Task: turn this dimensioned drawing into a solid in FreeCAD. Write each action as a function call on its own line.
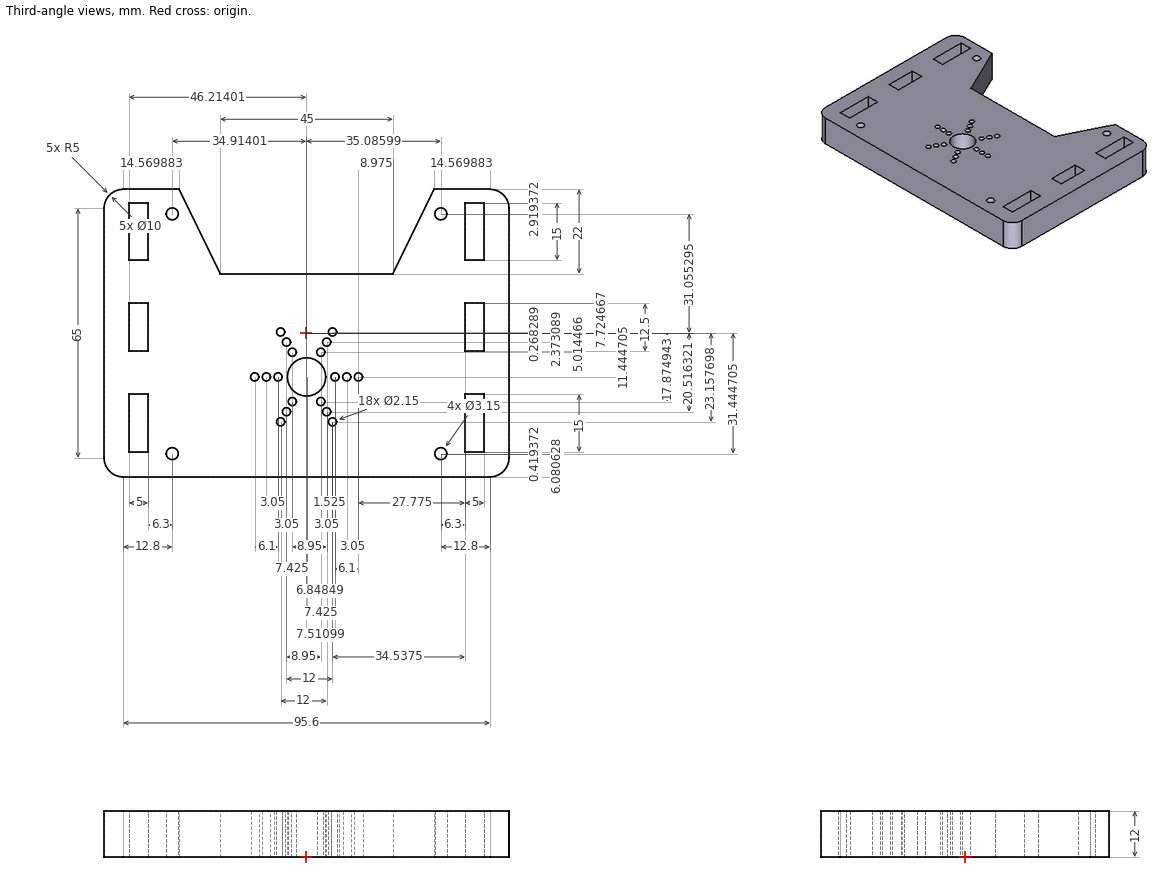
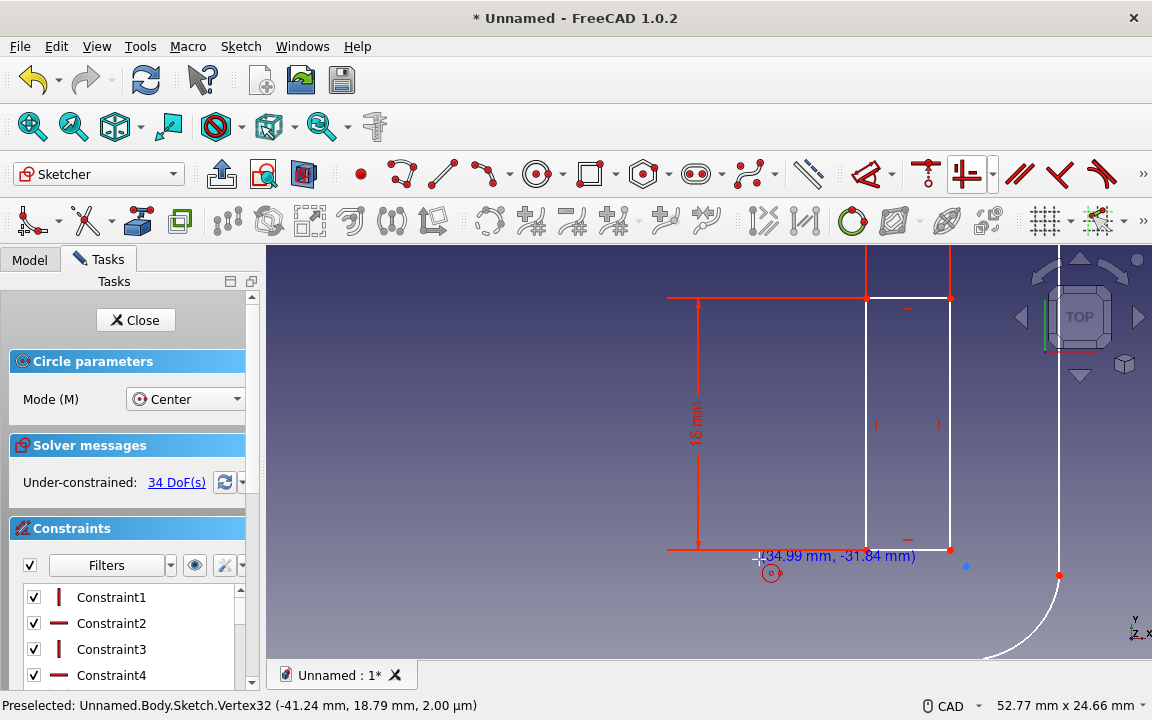
scroll(759, 560, down, 8)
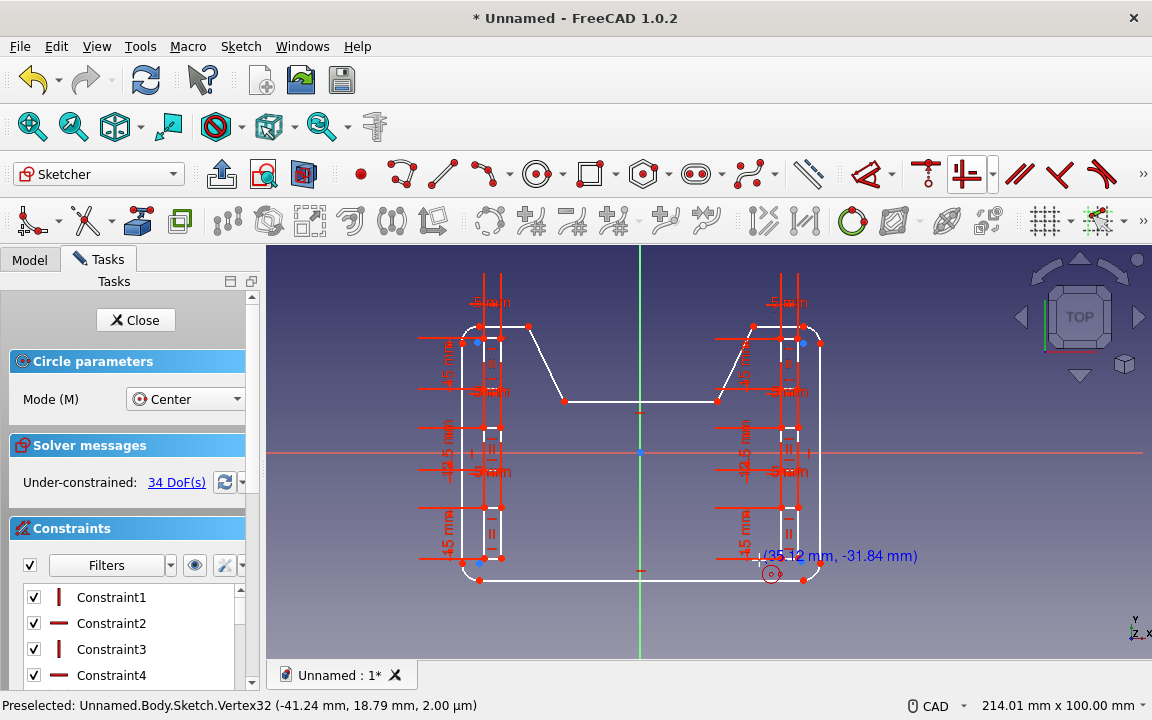
click(759, 559)
move(763, 556)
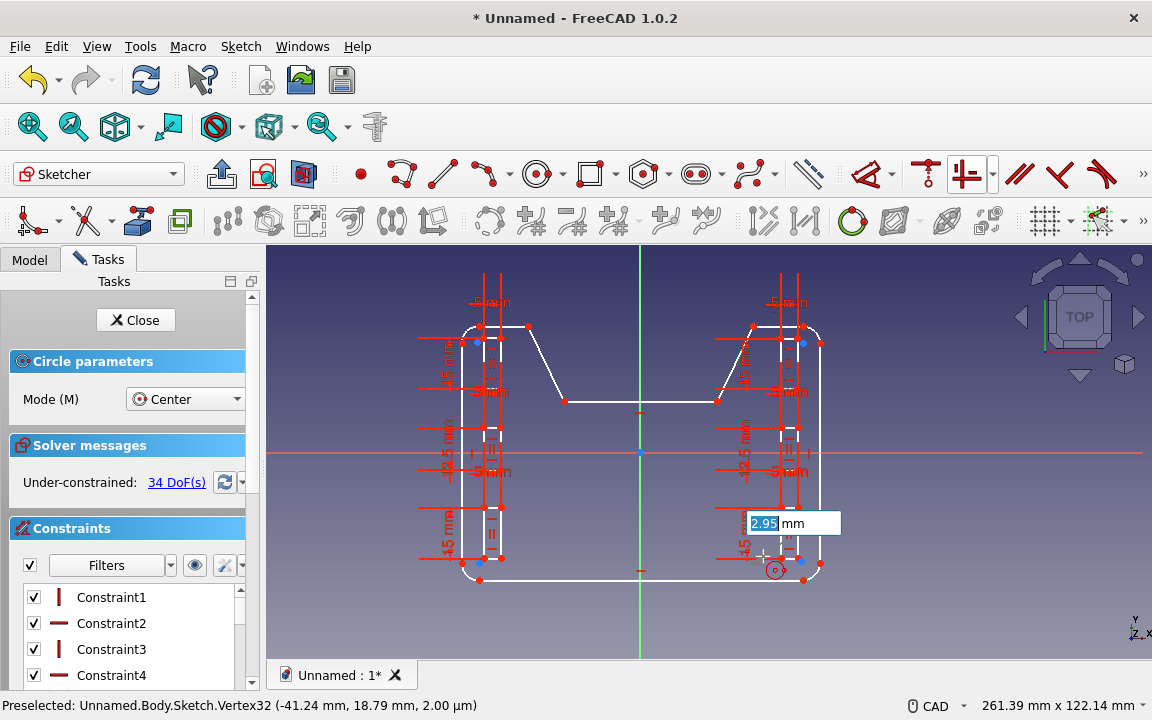
text(3.15)
key(Return)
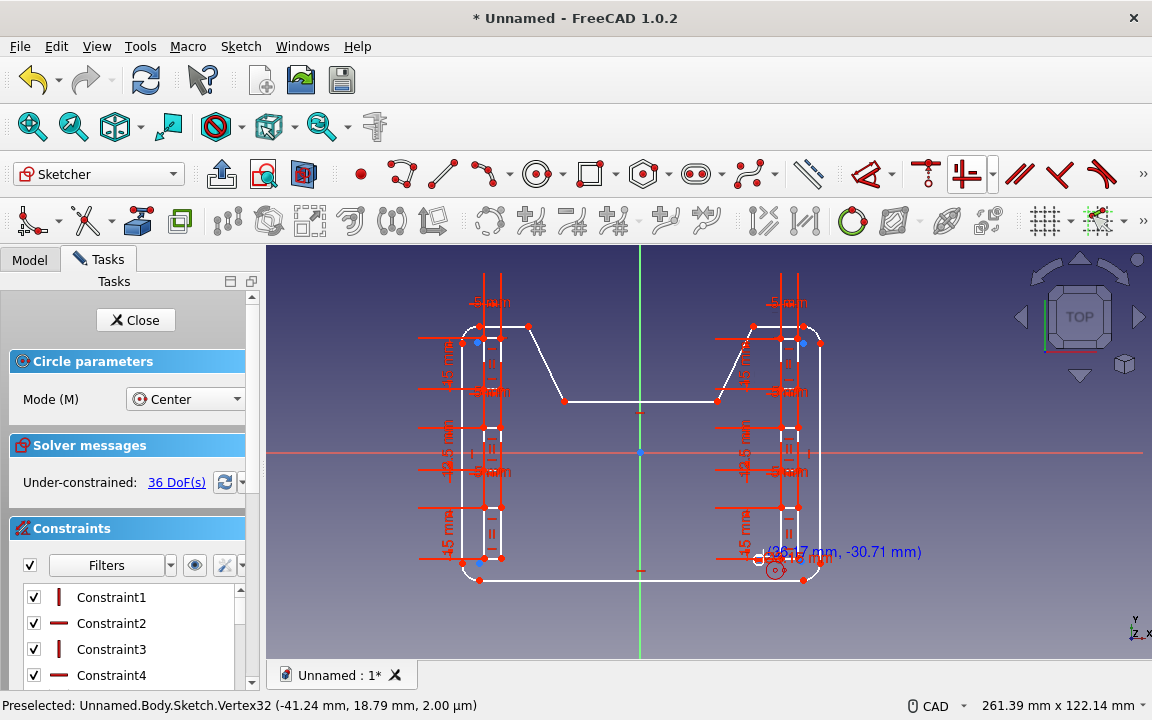
scroll(664, 531, up, 10)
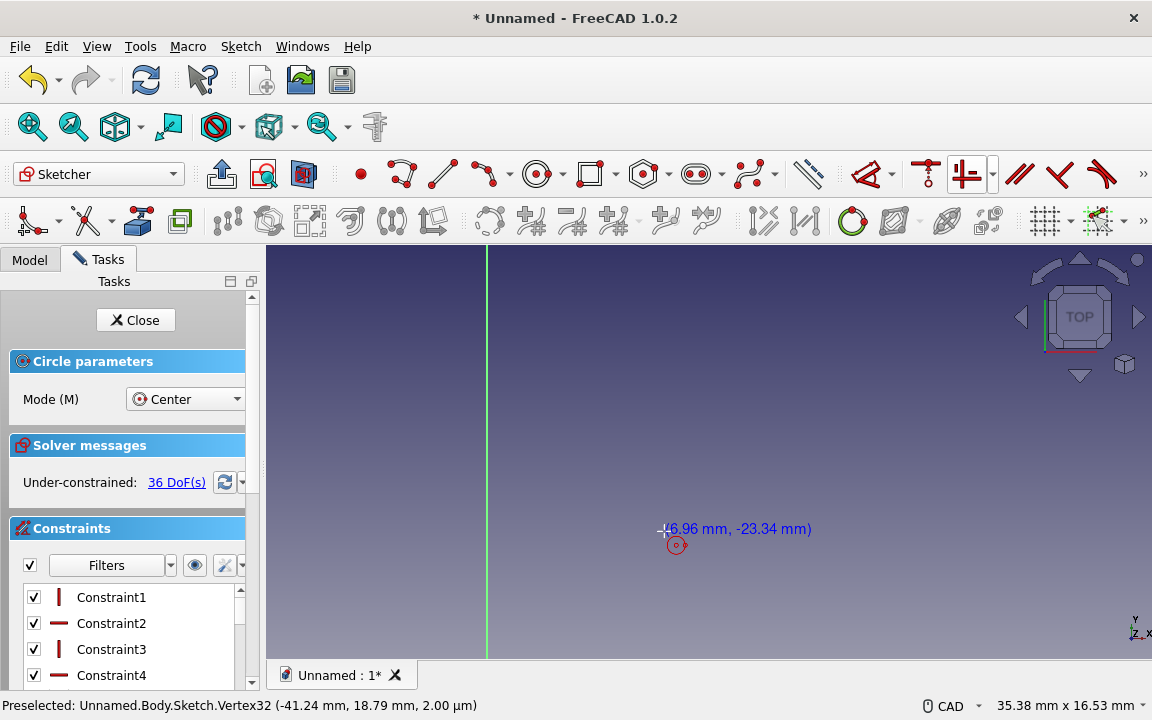
scroll(664, 531, down, 10)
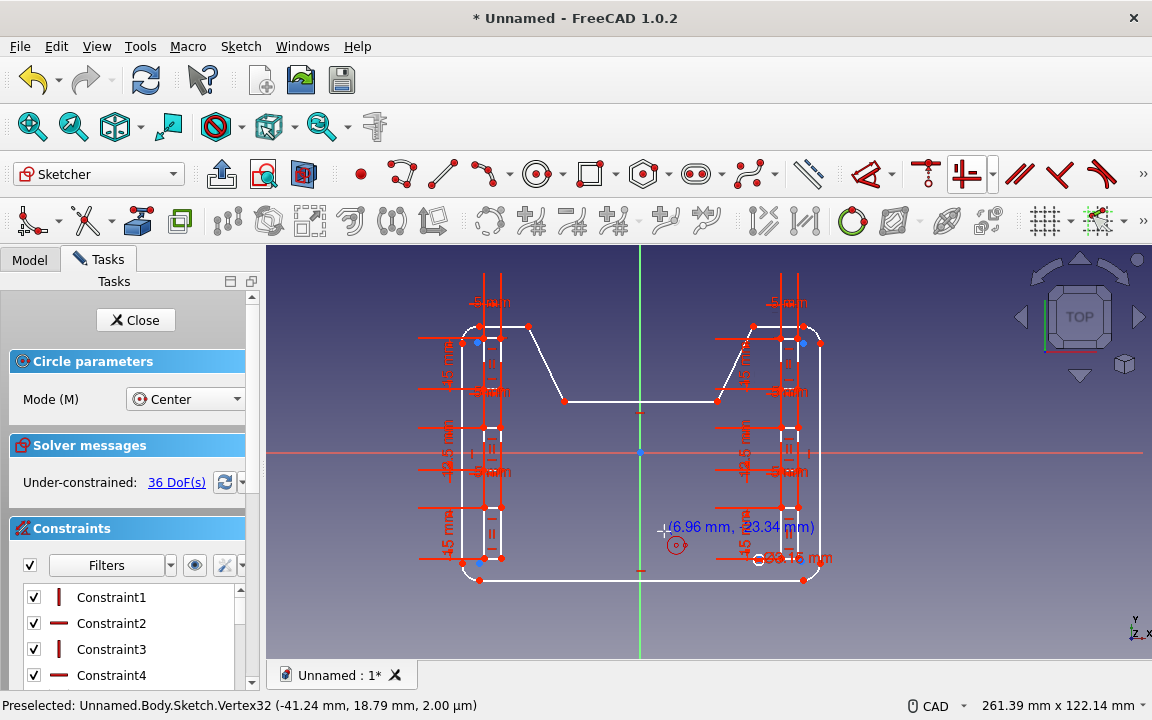
click(664, 531)
move(666, 529)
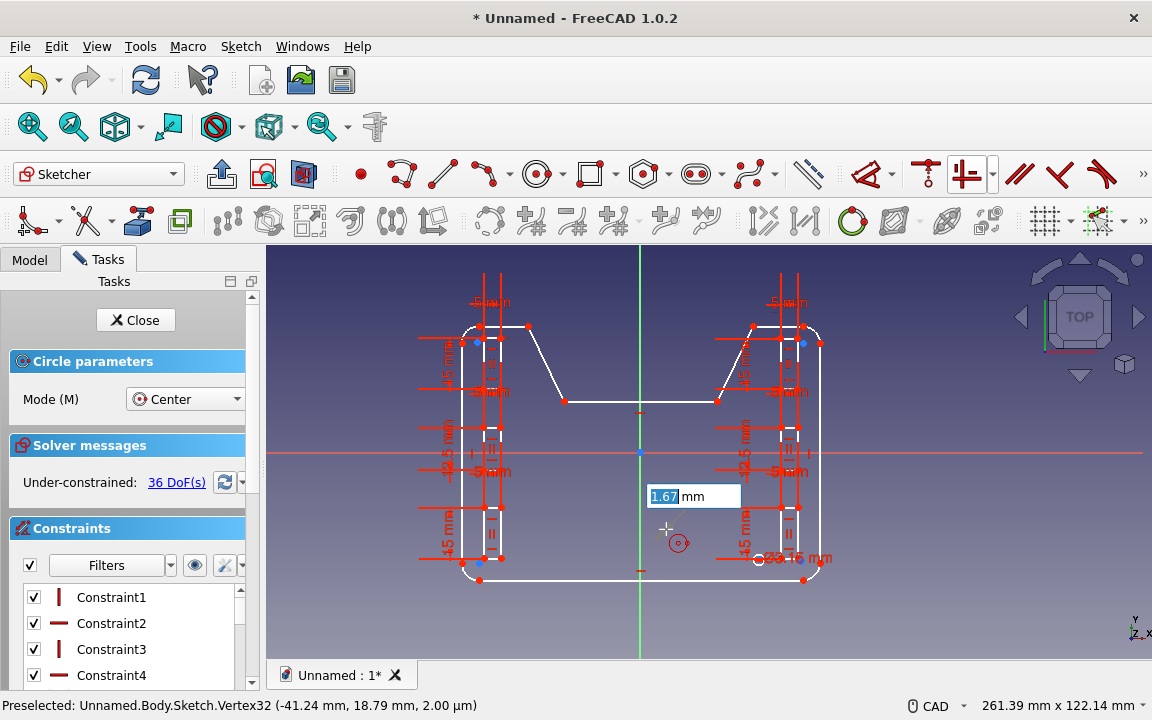
text(2.15)
key(Return)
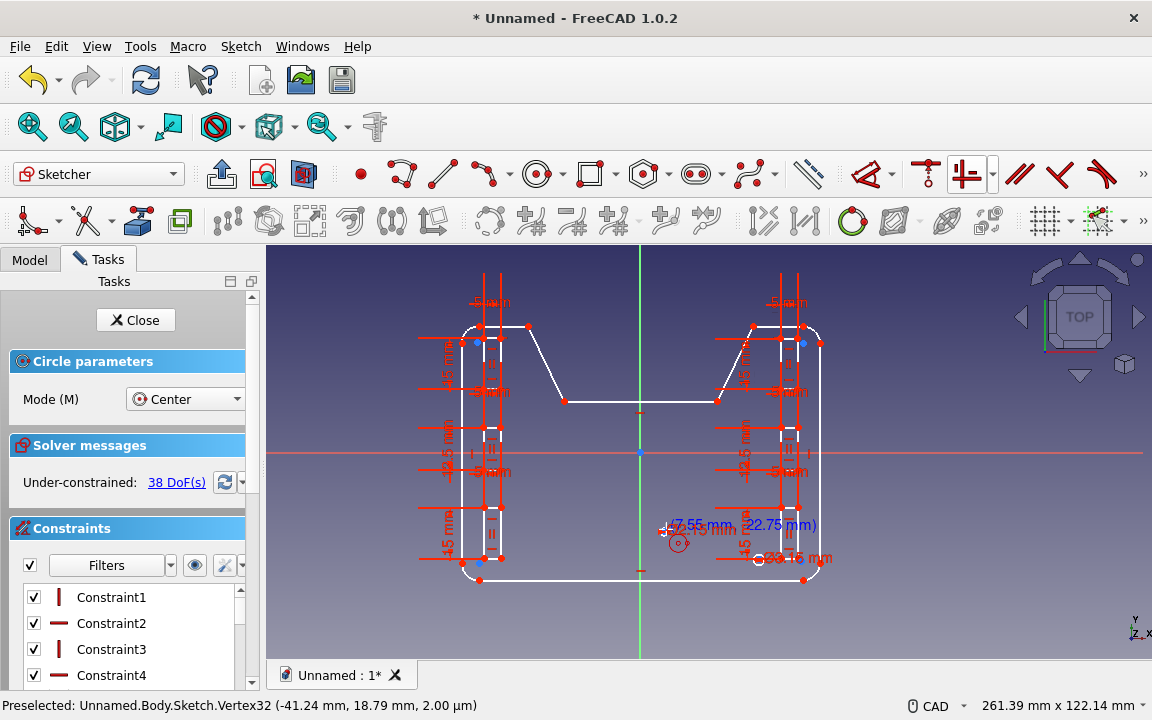
scroll(658, 522, up, 10)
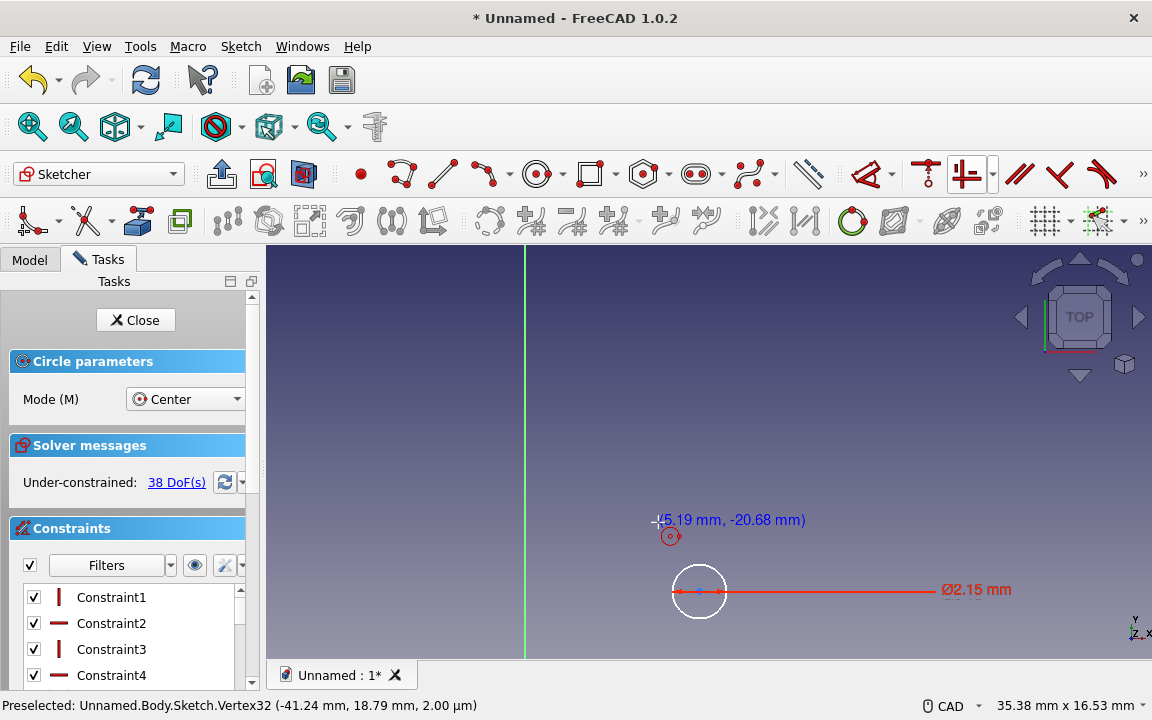
scroll(658, 522, down, 10)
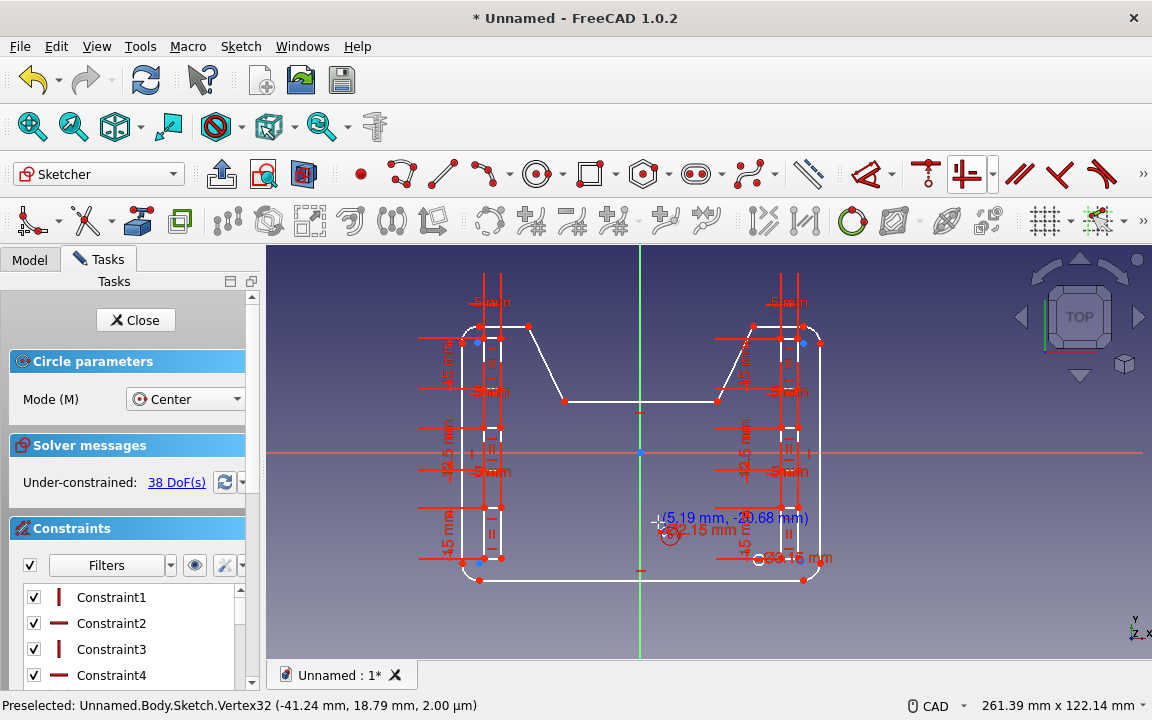
scroll(658, 522, up, 5)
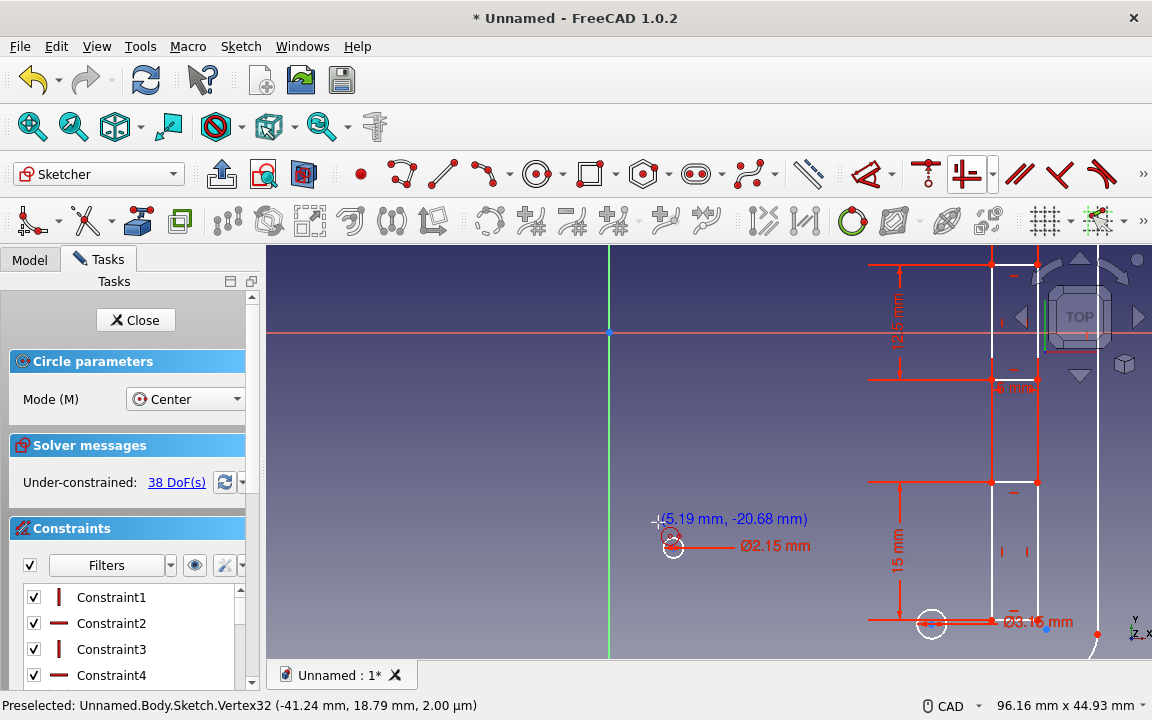
click(658, 522)
move(665, 515)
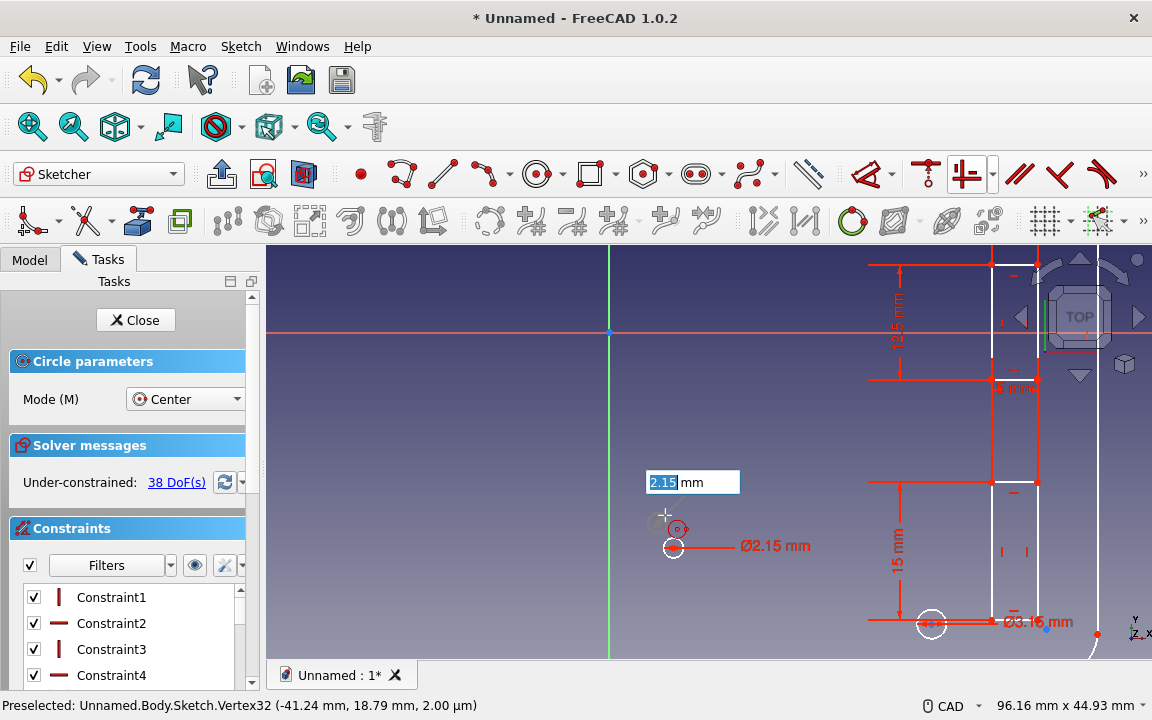
text(2.15)
key(Return)